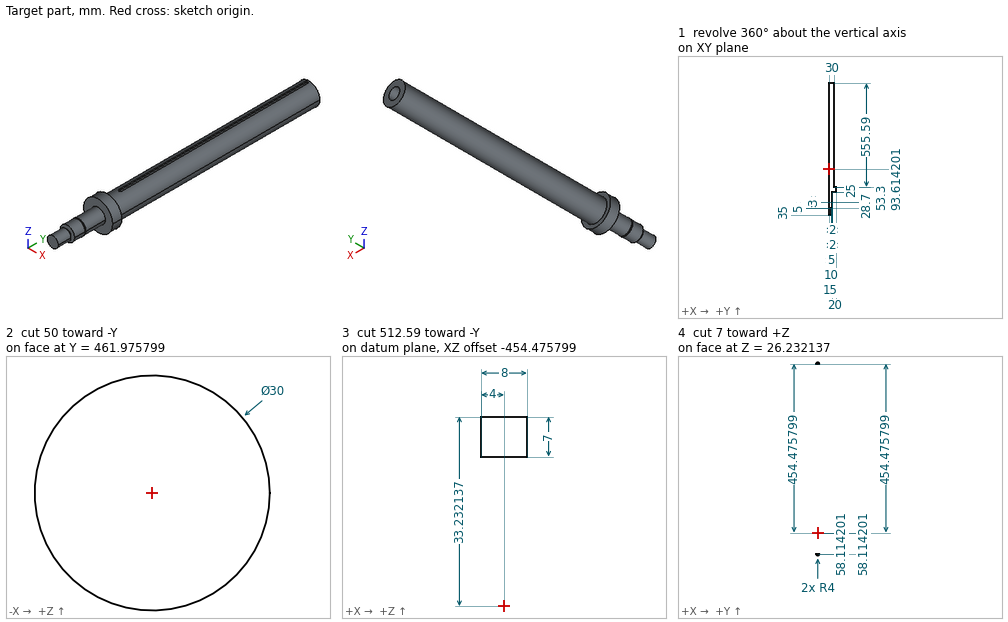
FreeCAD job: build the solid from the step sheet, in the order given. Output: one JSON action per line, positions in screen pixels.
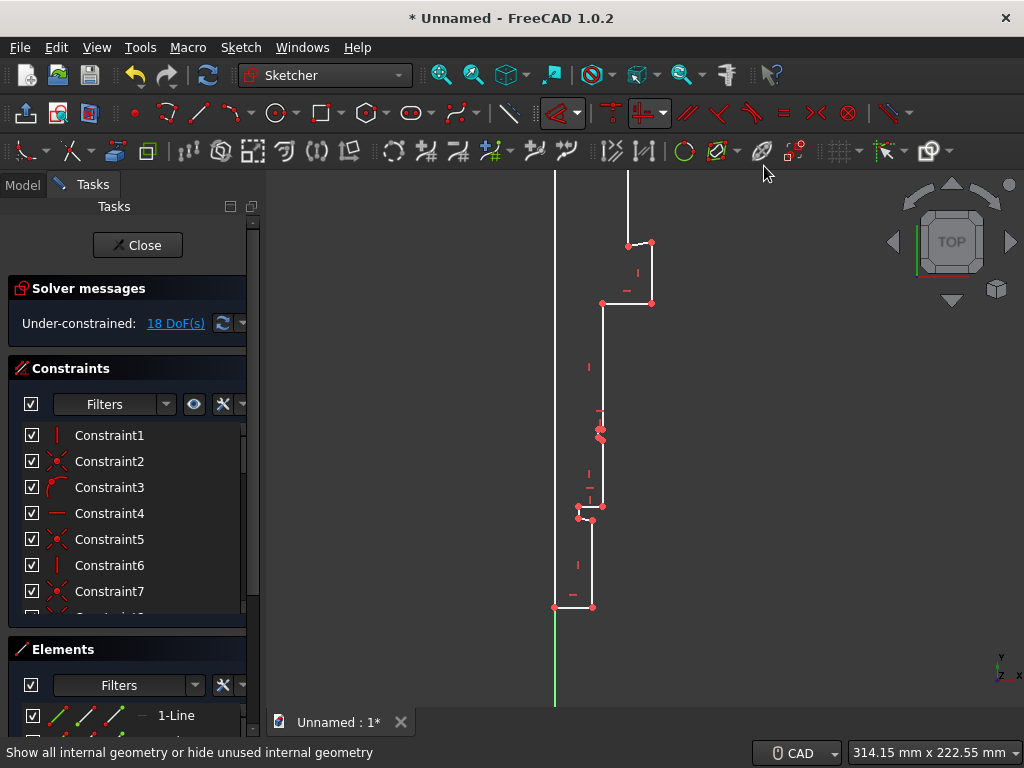
{"action": "scroll", "coordinate": [585, 520], "scroll_direction": "up", "scroll_amount": 4}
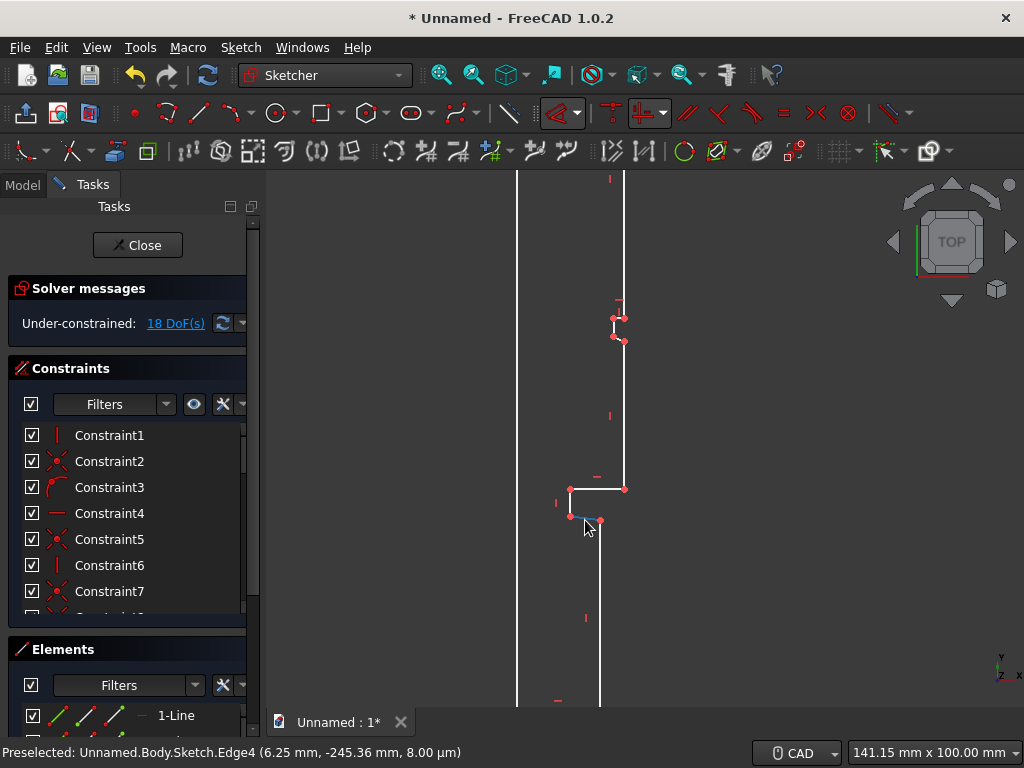
{"action": "left_click", "coordinate": [585, 518]}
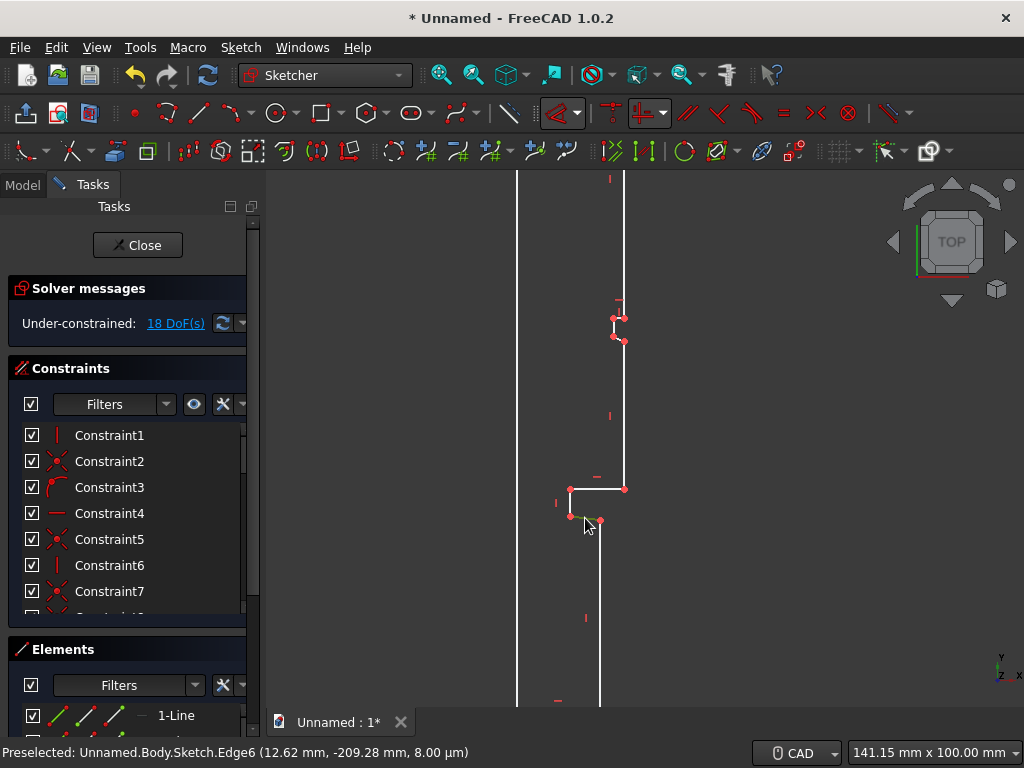
{"action": "key", "text": "h"}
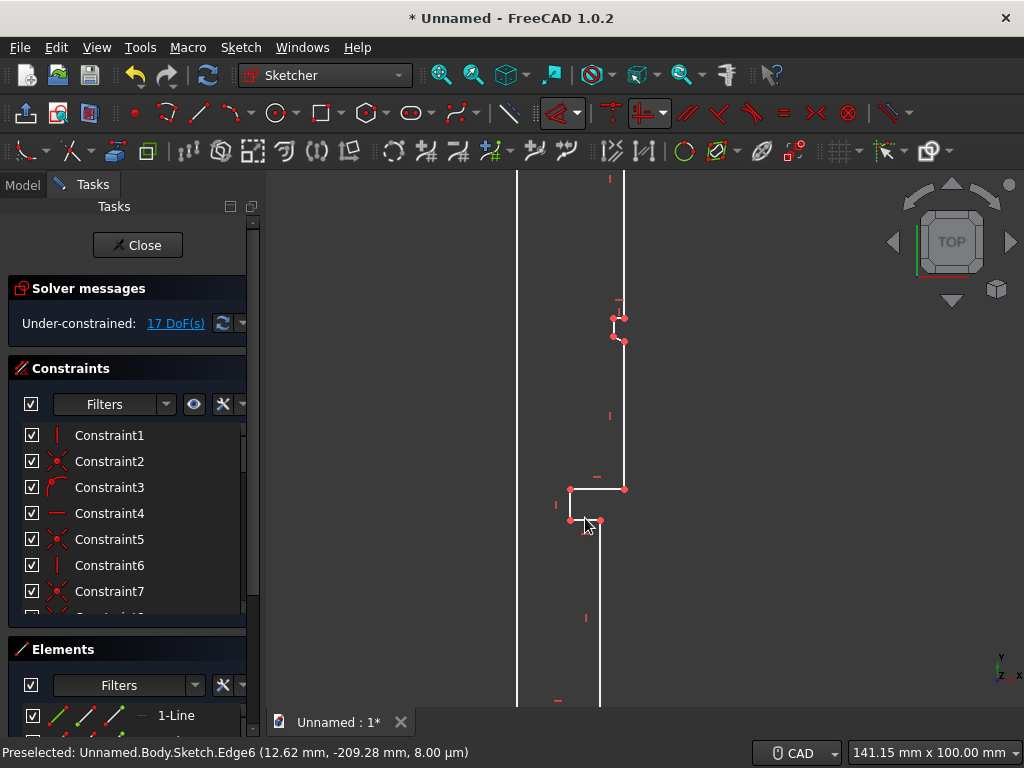
{"action": "scroll", "coordinate": [619, 339], "scroll_direction": "up", "scroll_amount": 2}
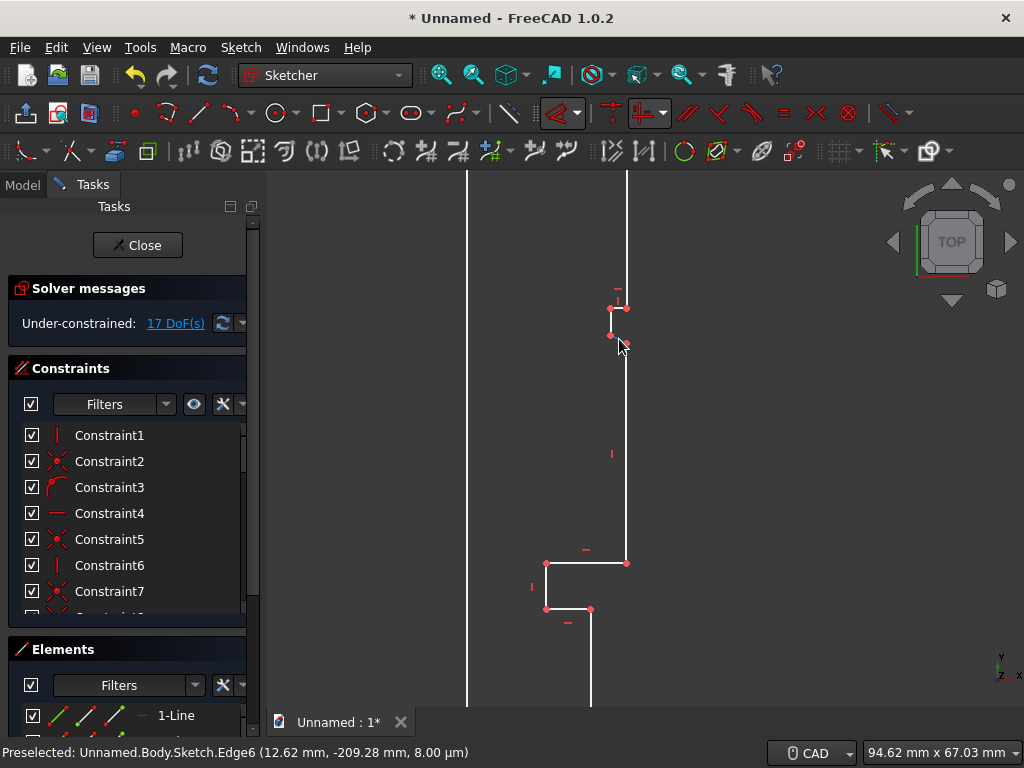
{"action": "left_click", "coordinate": [619, 339]}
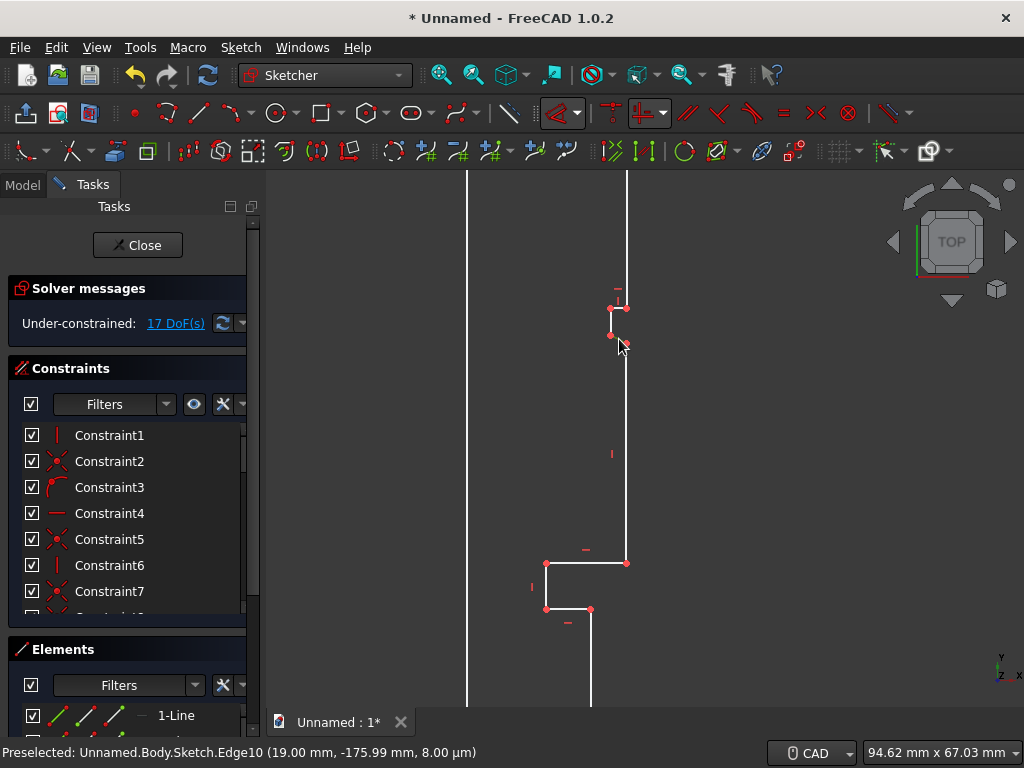
{"action": "key", "text": "h"}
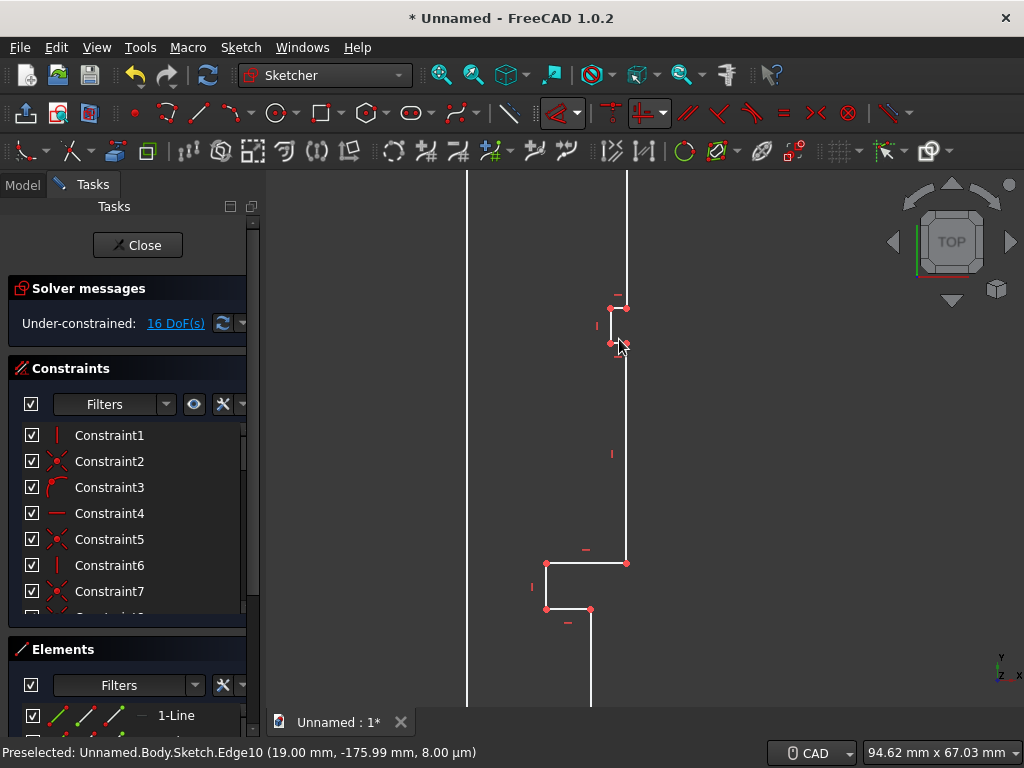
{"action": "scroll", "coordinate": [573, 593], "scroll_direction": "down", "scroll_amount": 14}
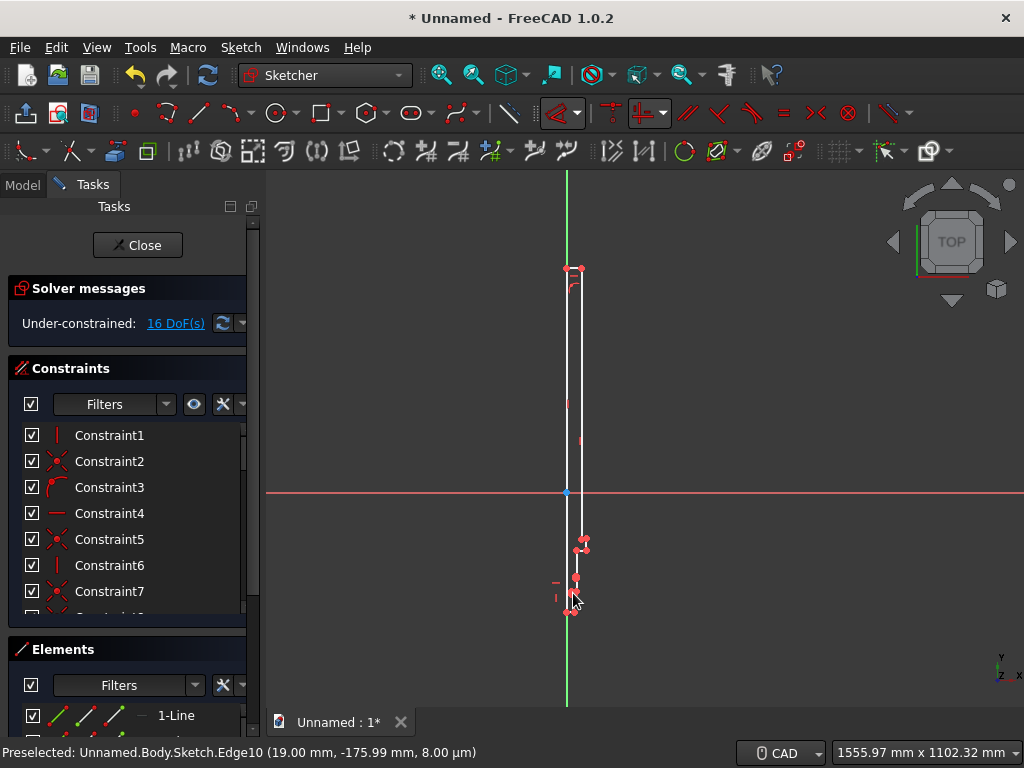
{"action": "scroll", "coordinate": [585, 539], "scroll_direction": "up", "scroll_amount": 12}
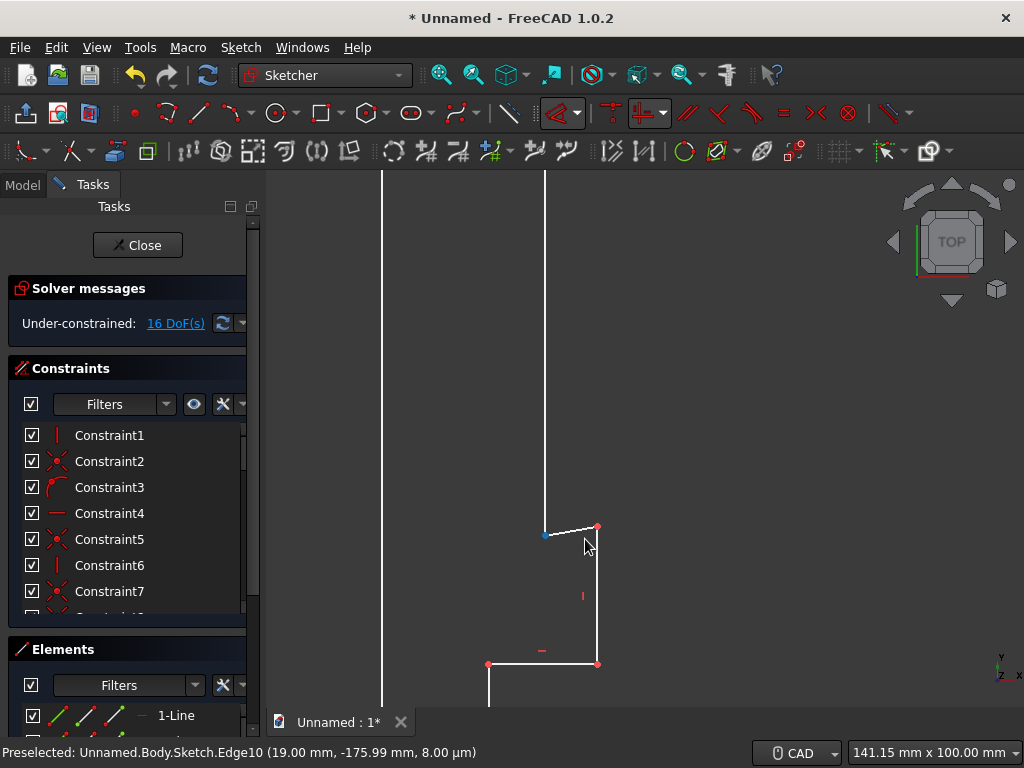
{"action": "left_click", "coordinate": [582, 530]}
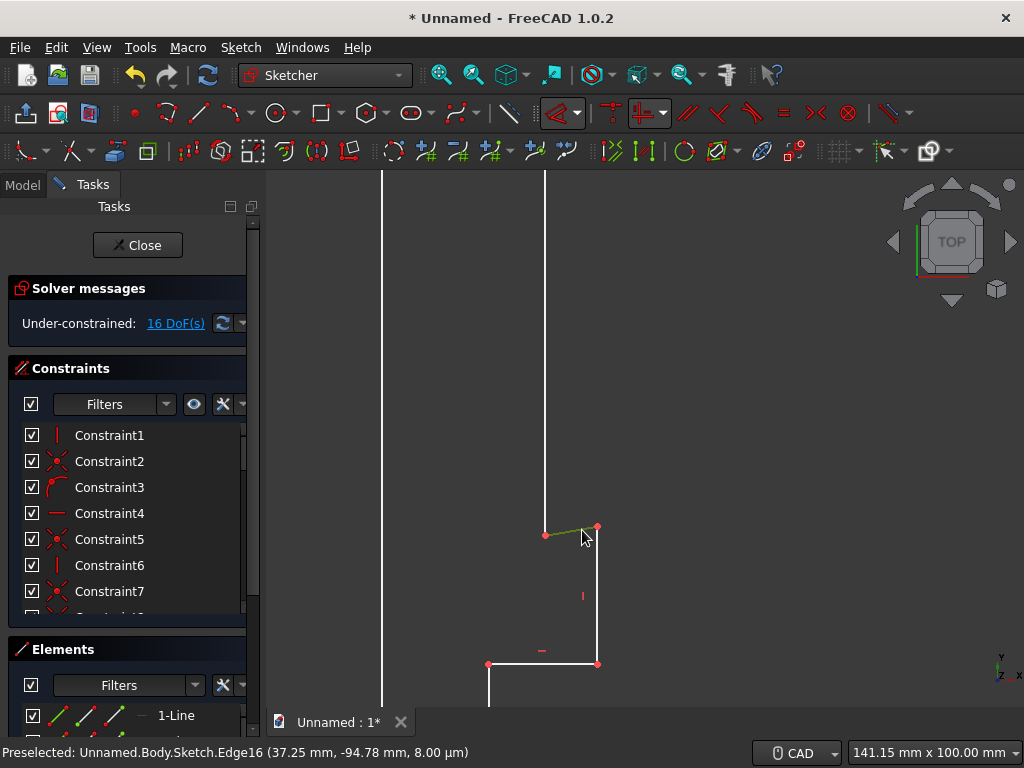
{"action": "key", "text": "h"}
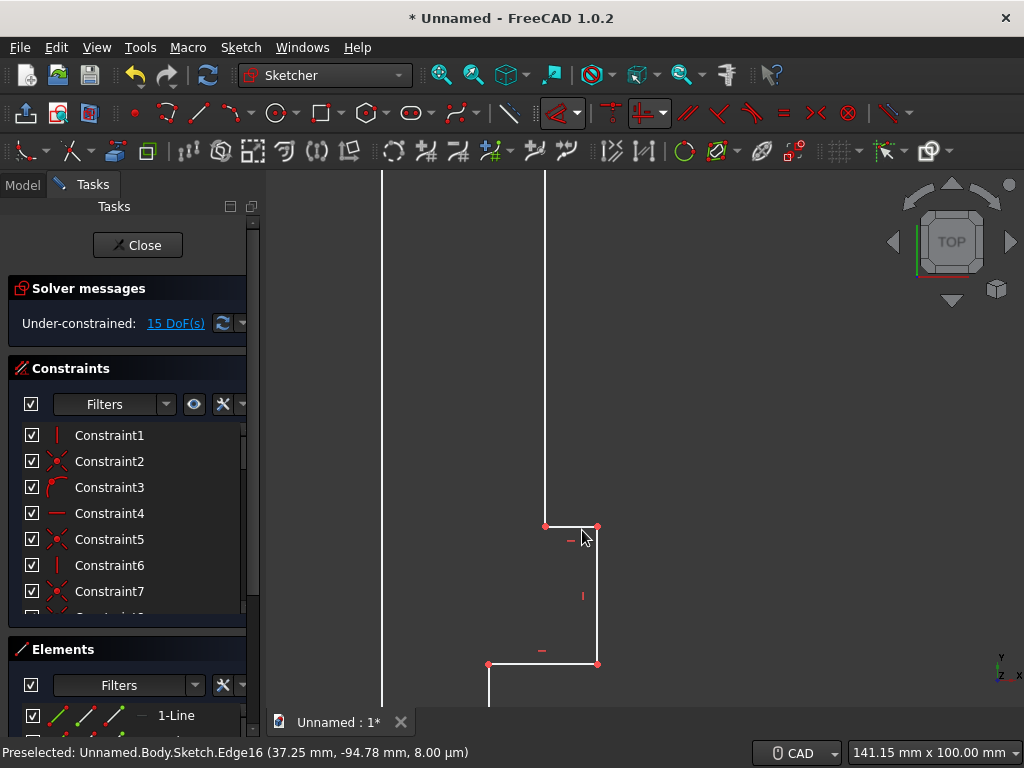
{"action": "key", "text": "d"}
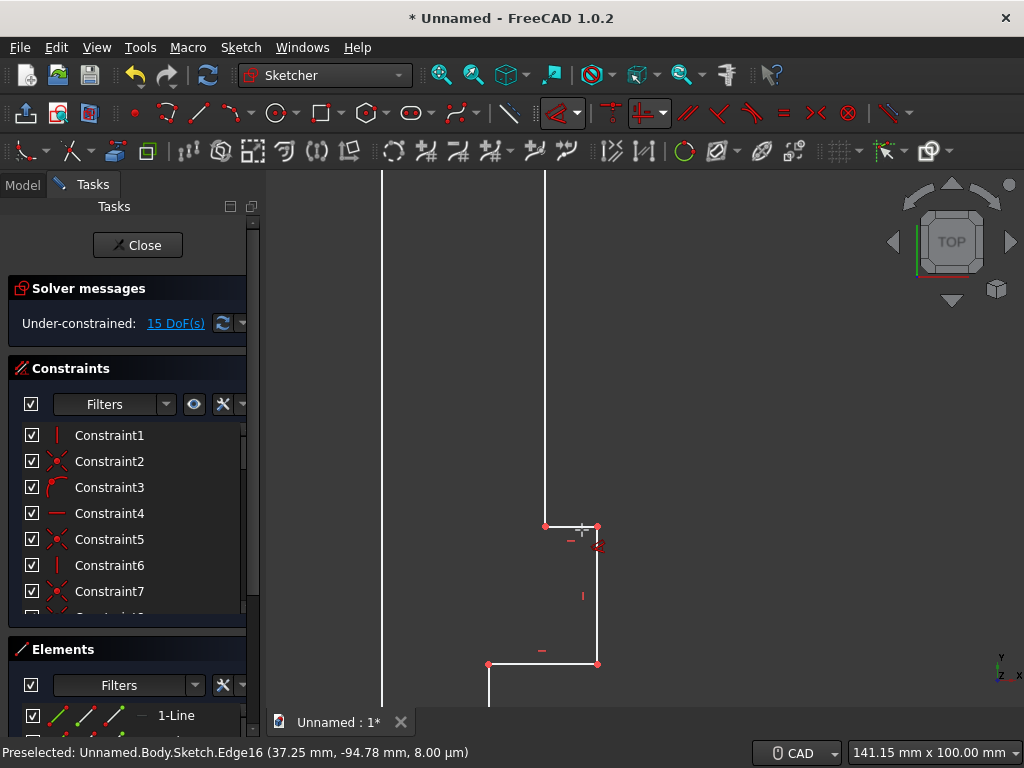
{"action": "scroll", "coordinate": [585, 539], "scroll_direction": "down", "scroll_amount": 12}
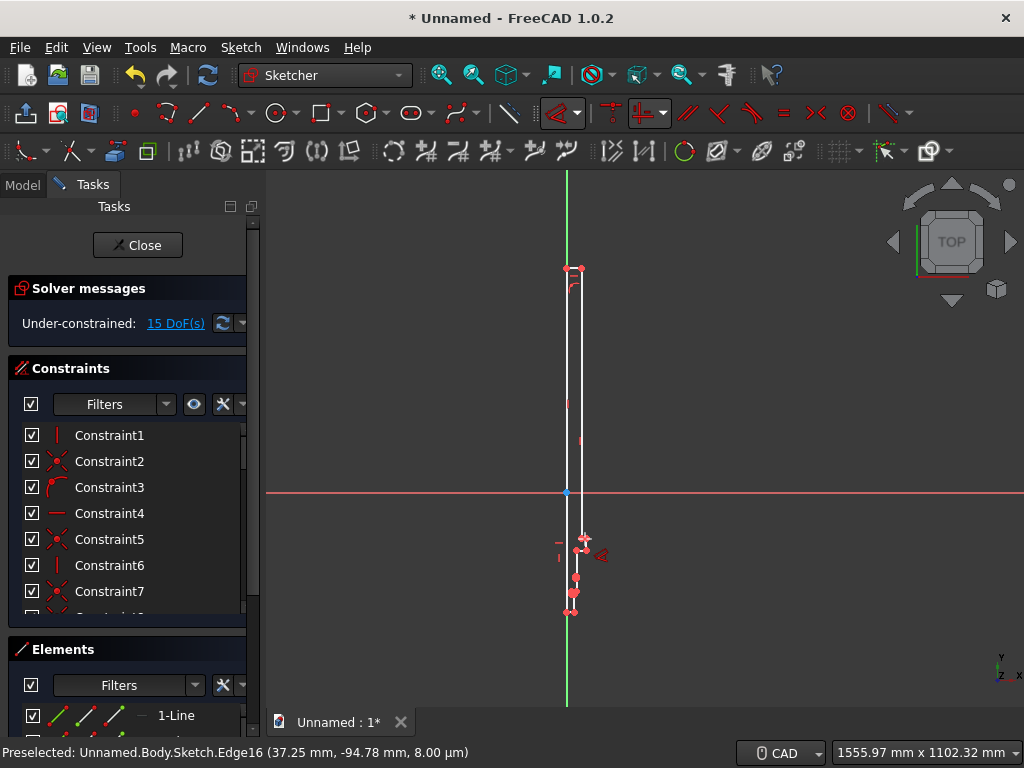
{"action": "scroll", "coordinate": [573, 595], "scroll_direction": "up", "scroll_amount": 14}